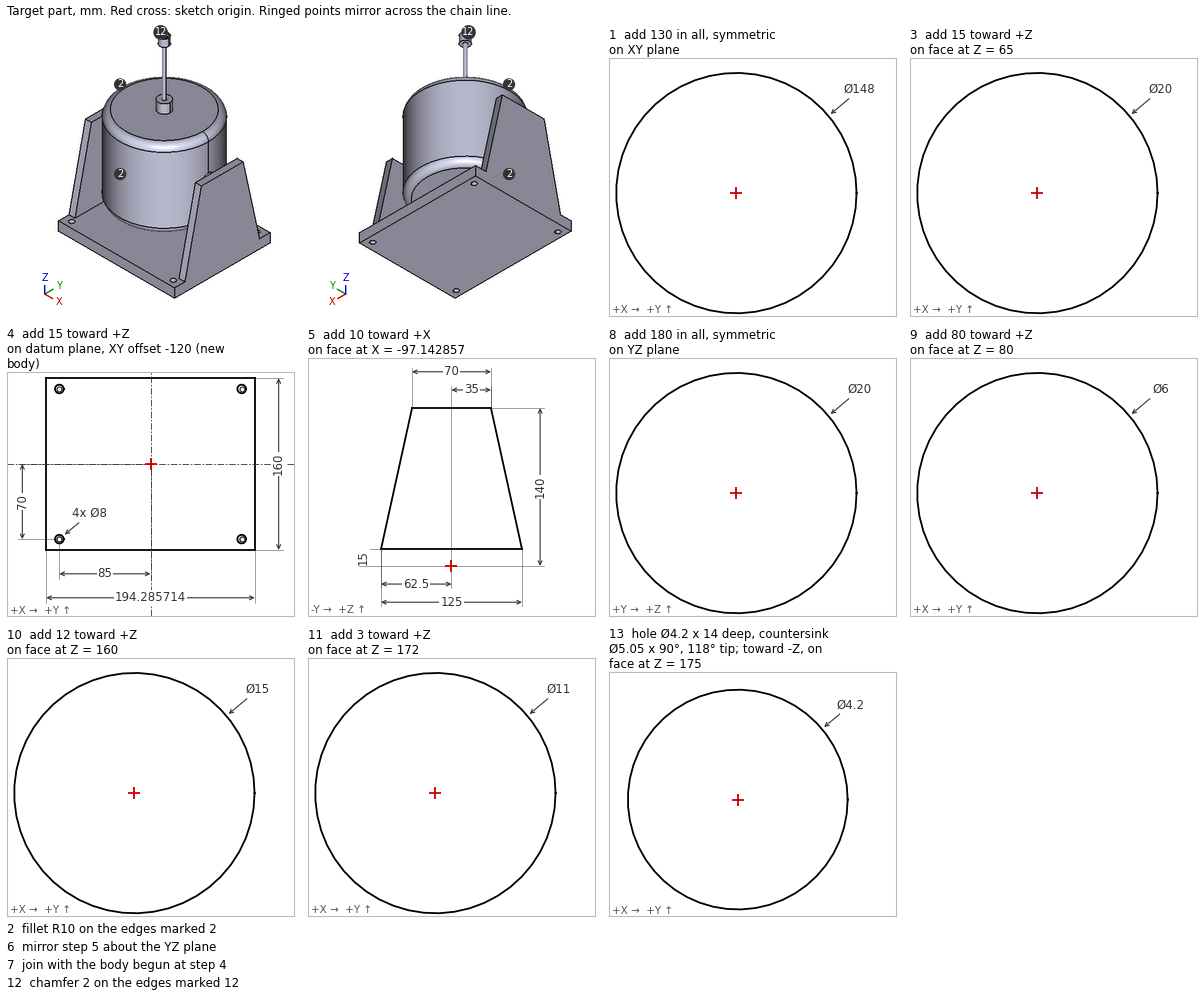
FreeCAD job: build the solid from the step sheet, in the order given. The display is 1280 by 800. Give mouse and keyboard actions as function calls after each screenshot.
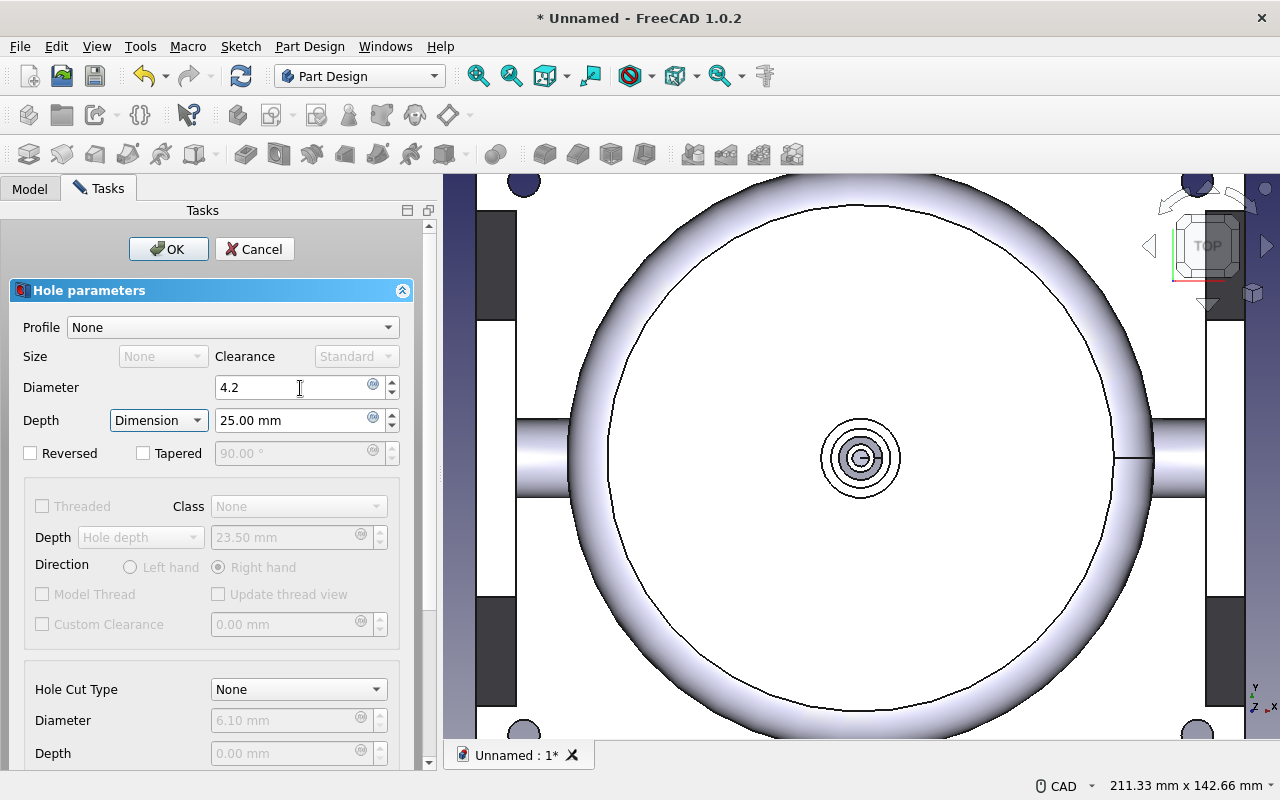
triple_click(300, 420)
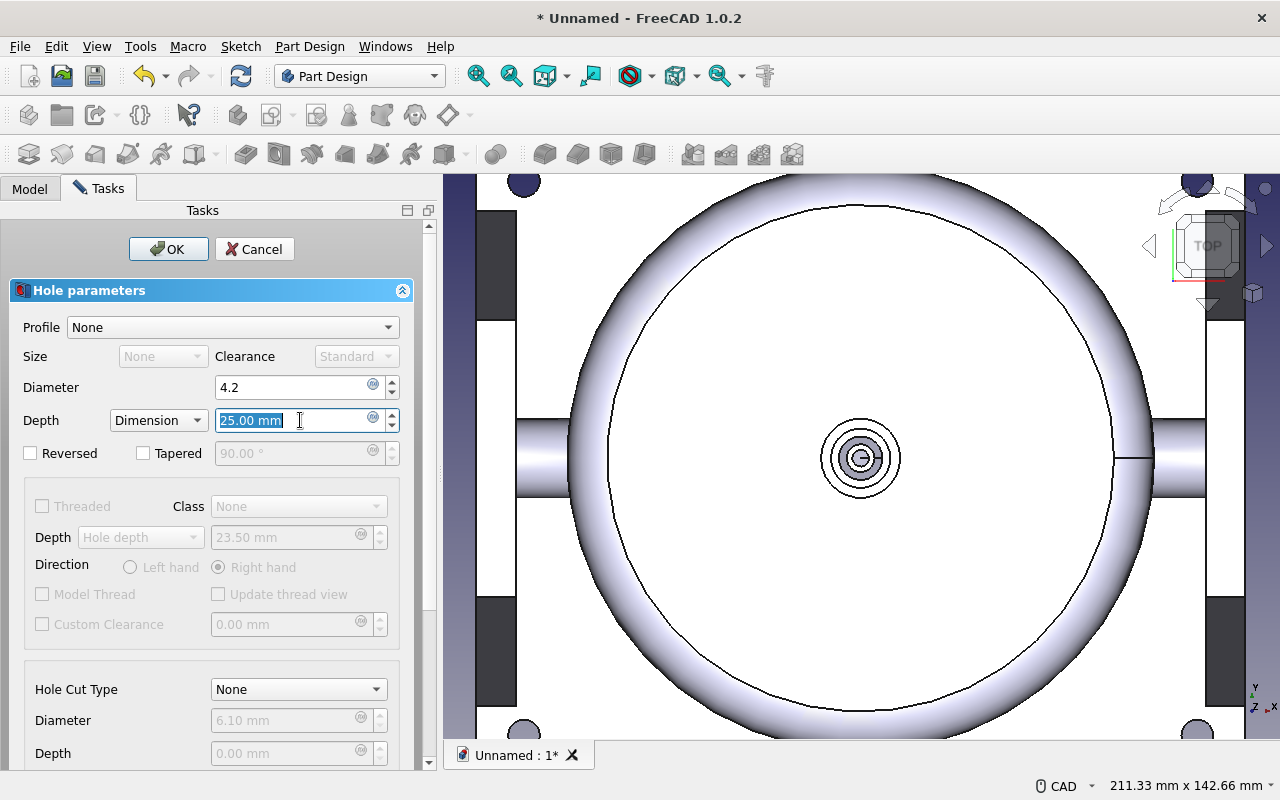
text(14)
key(Tab)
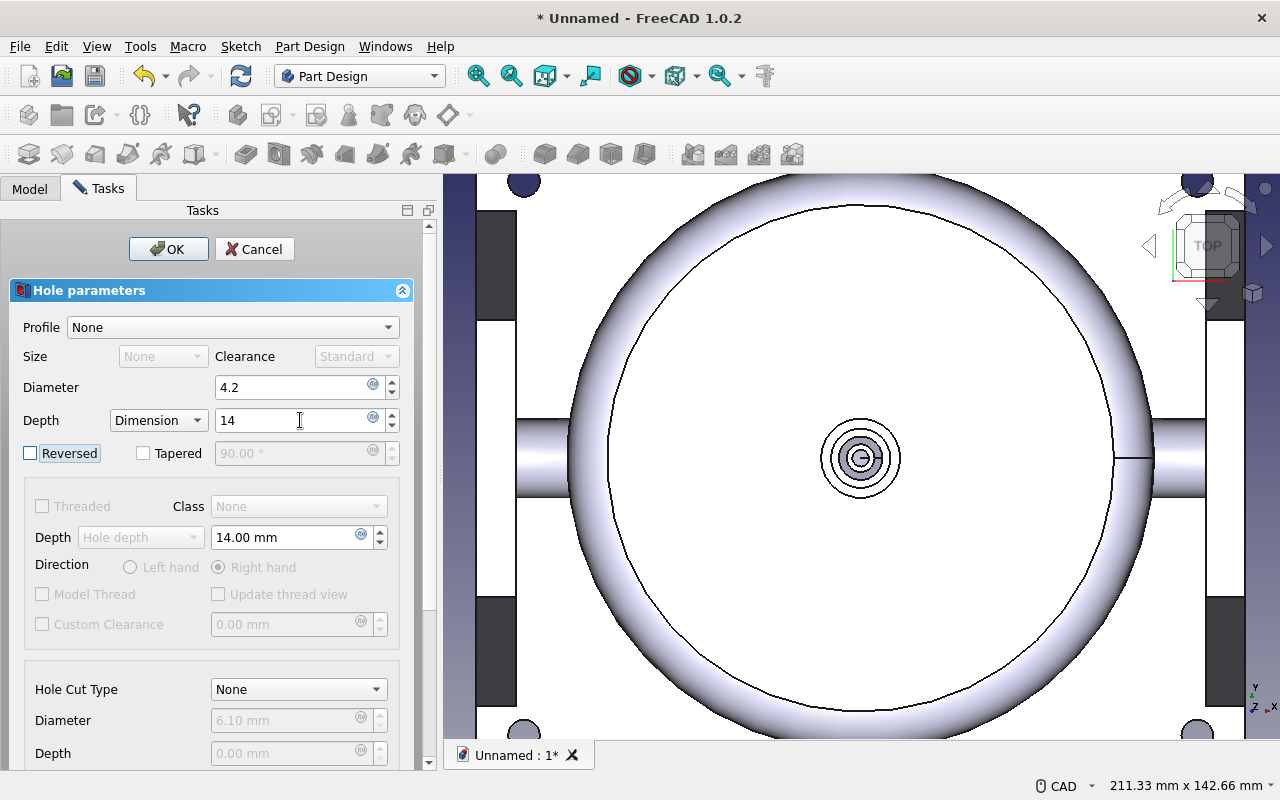
click(300, 690)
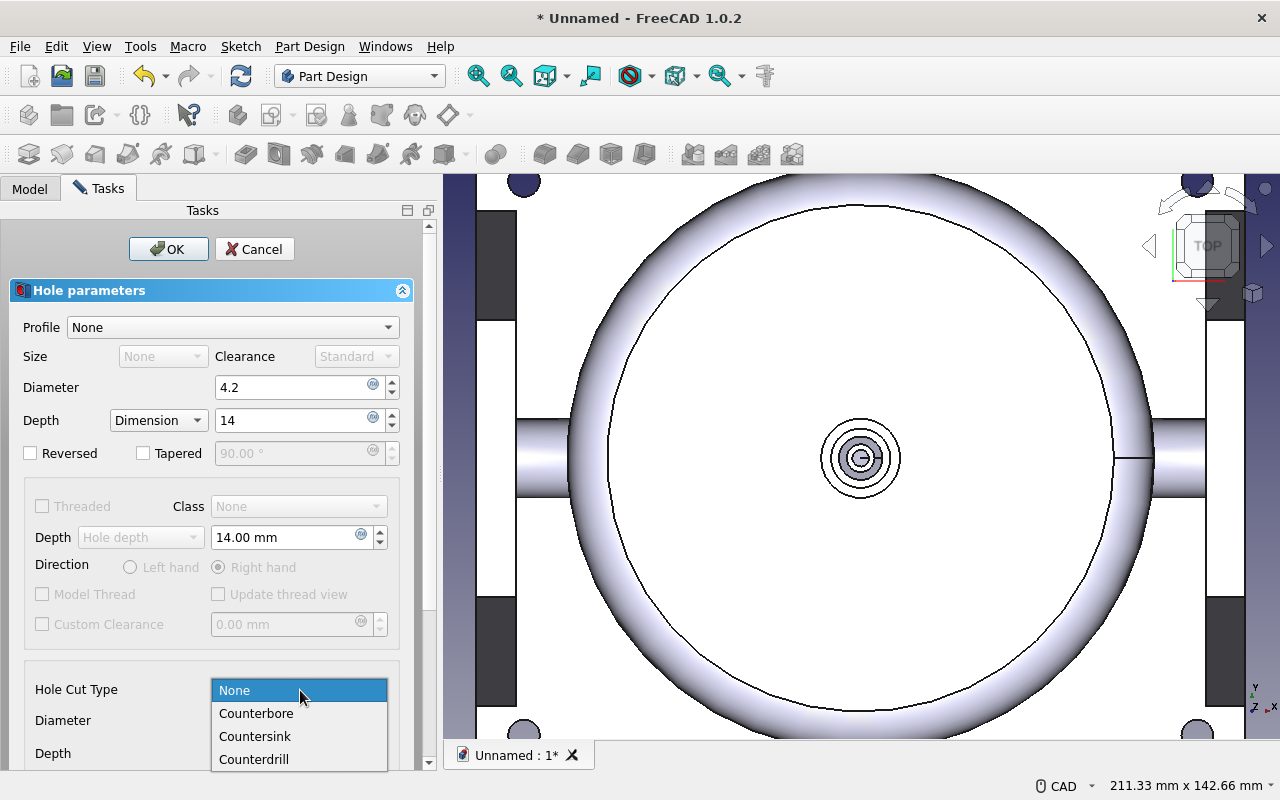
click(298, 736)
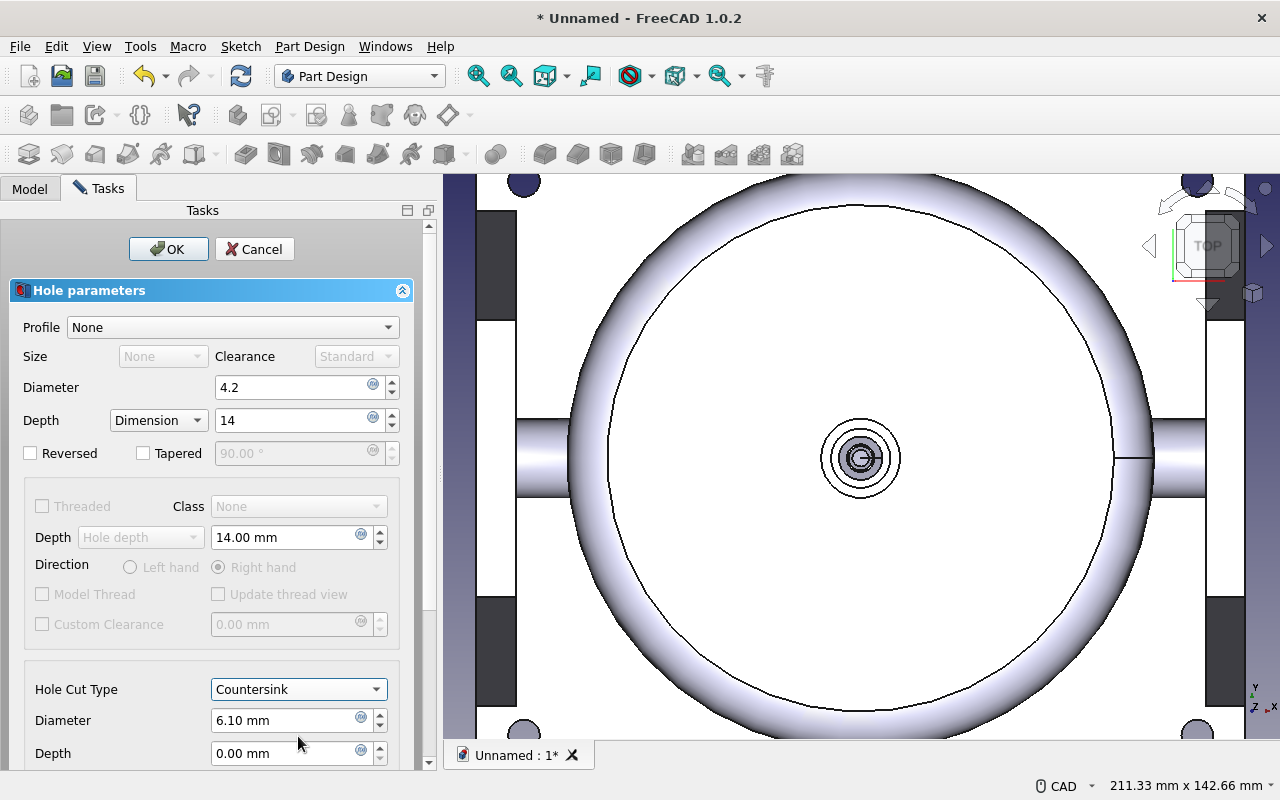
triple_click(292, 720)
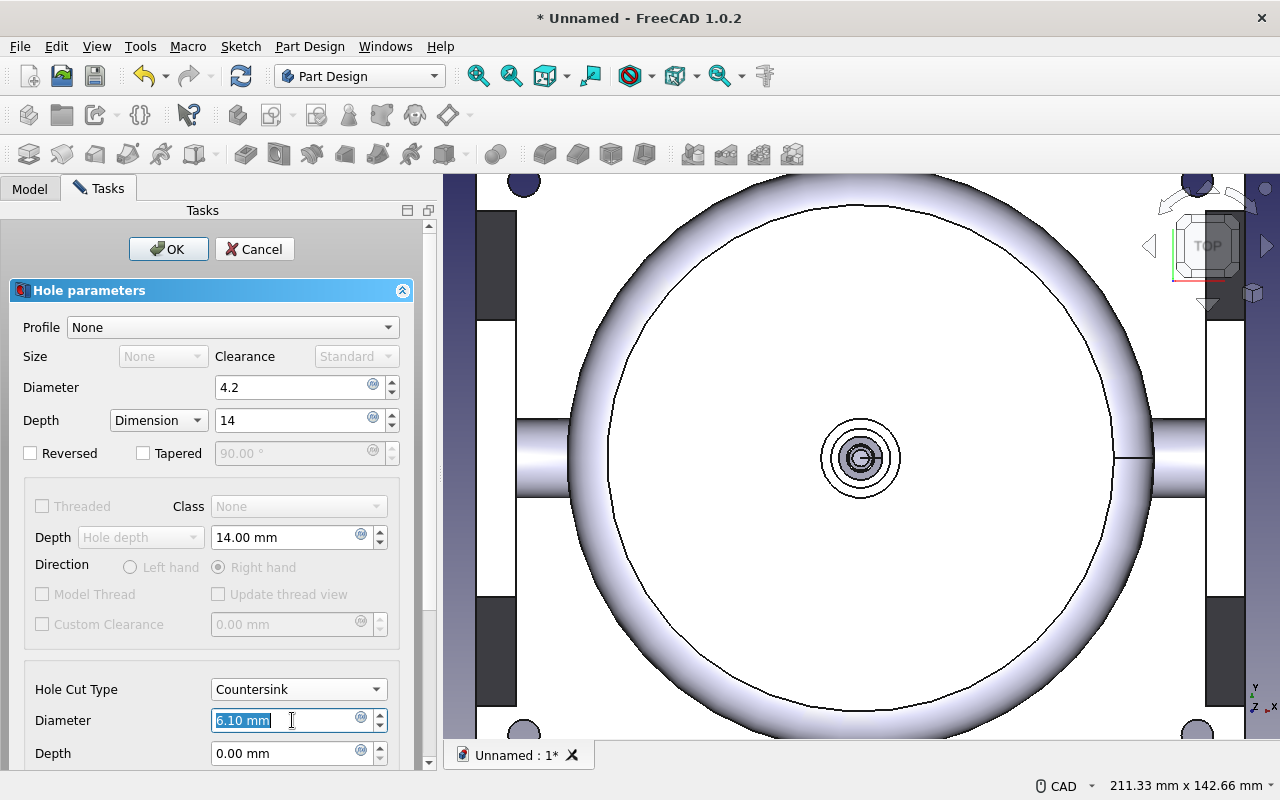
text(5.05)
key(Tab)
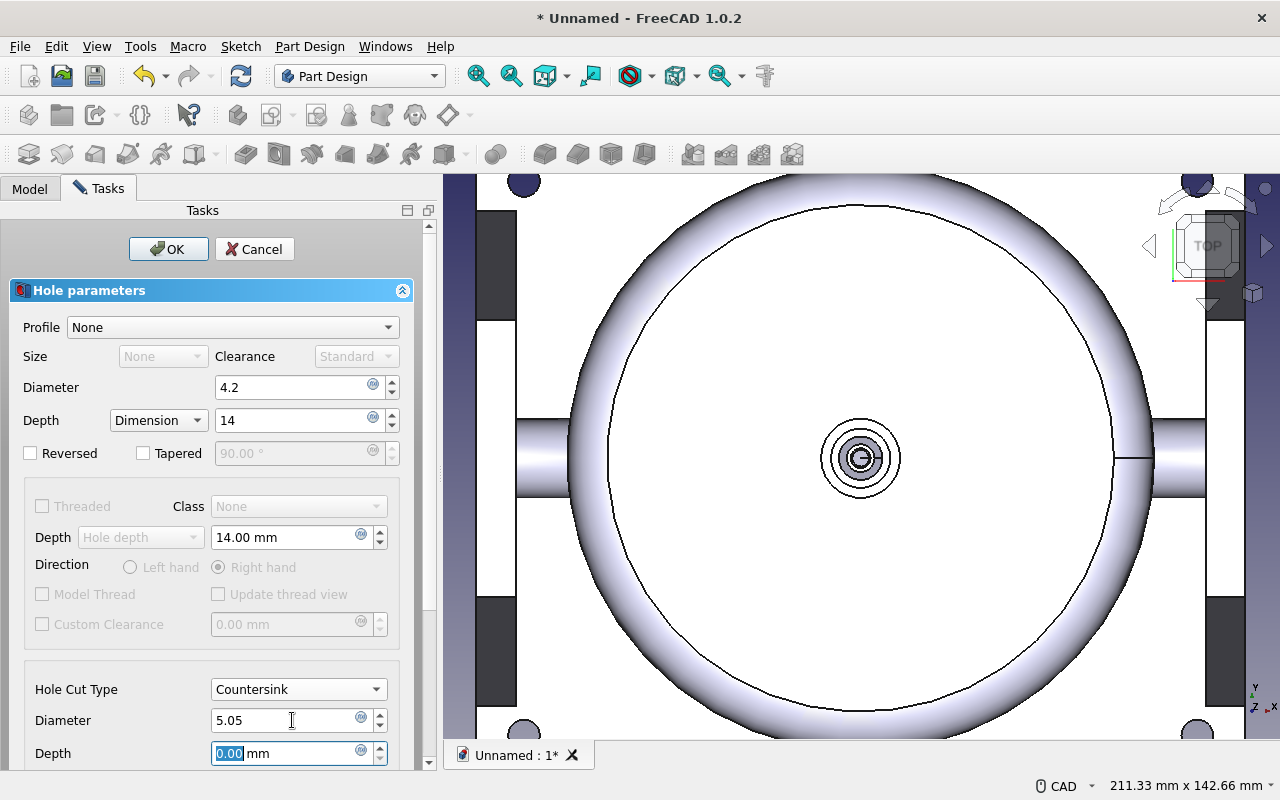
click(169, 249)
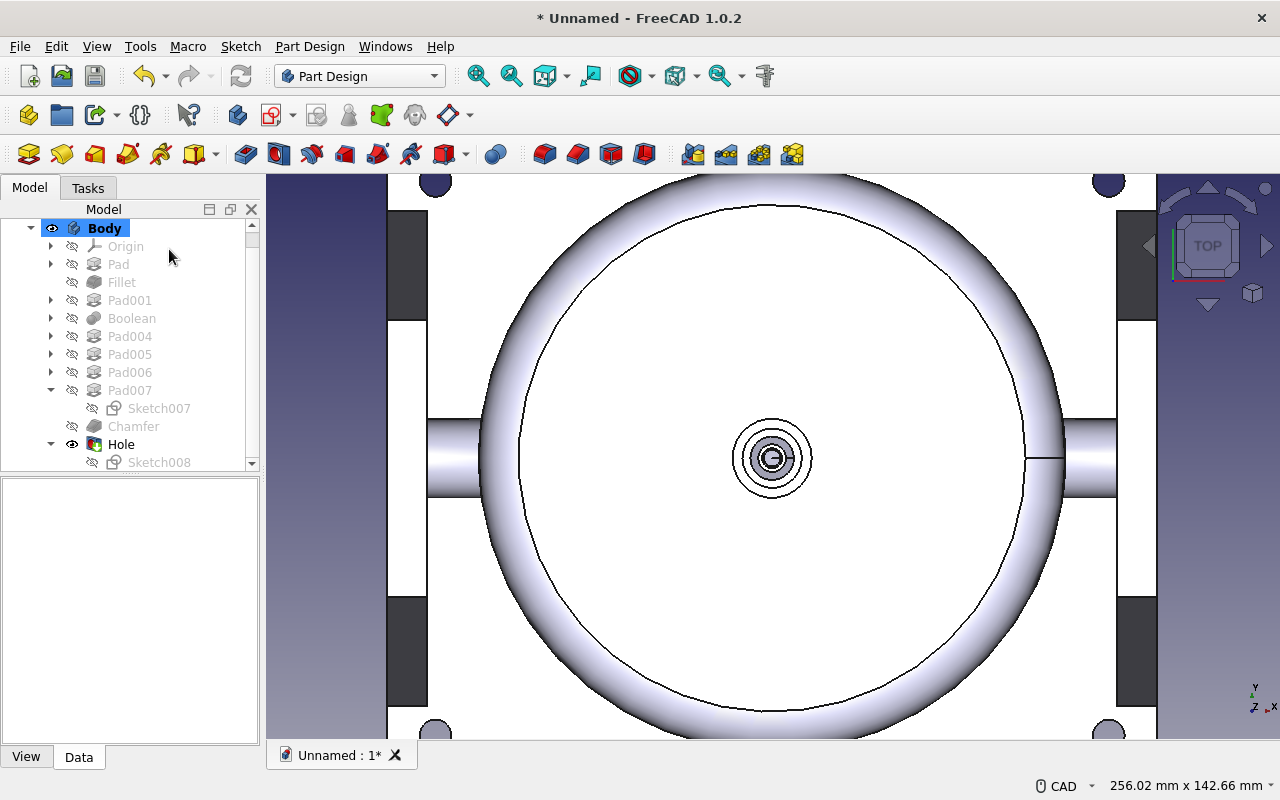
key(0)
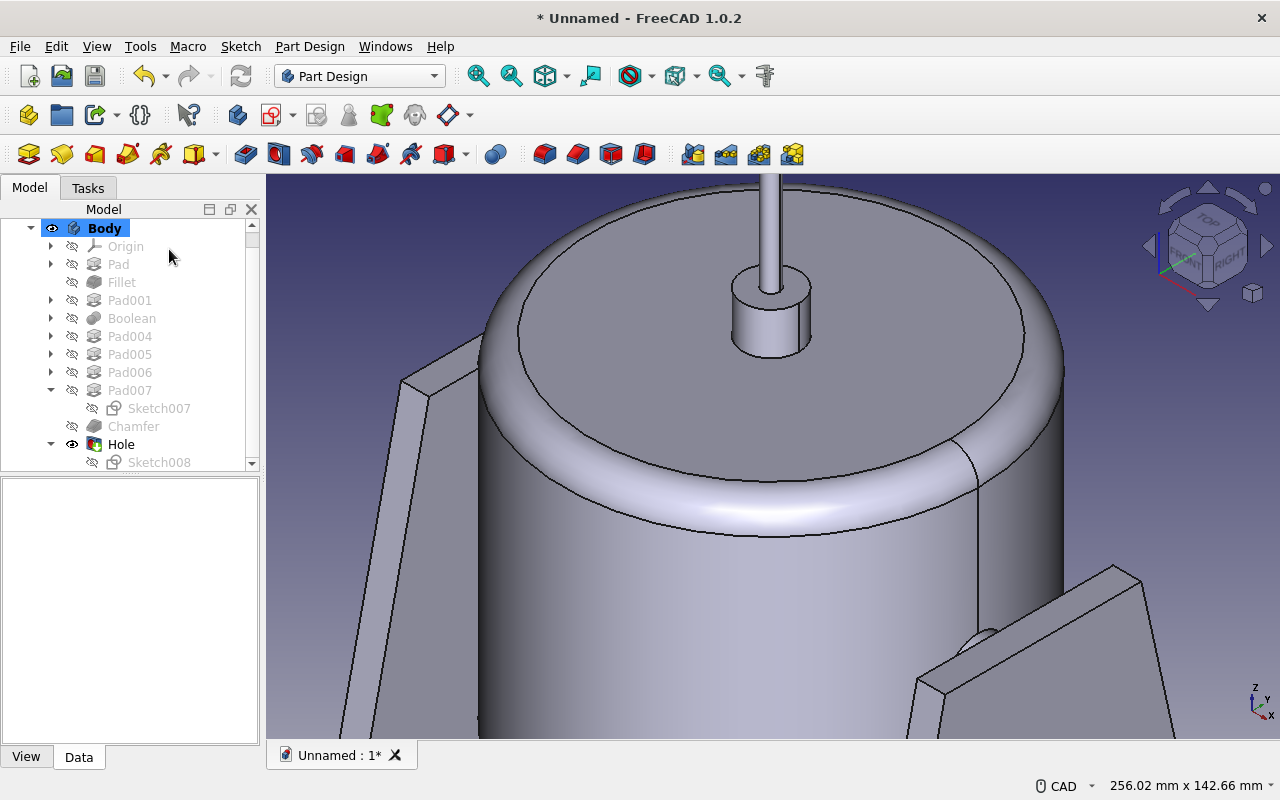
key(v)
key(f)